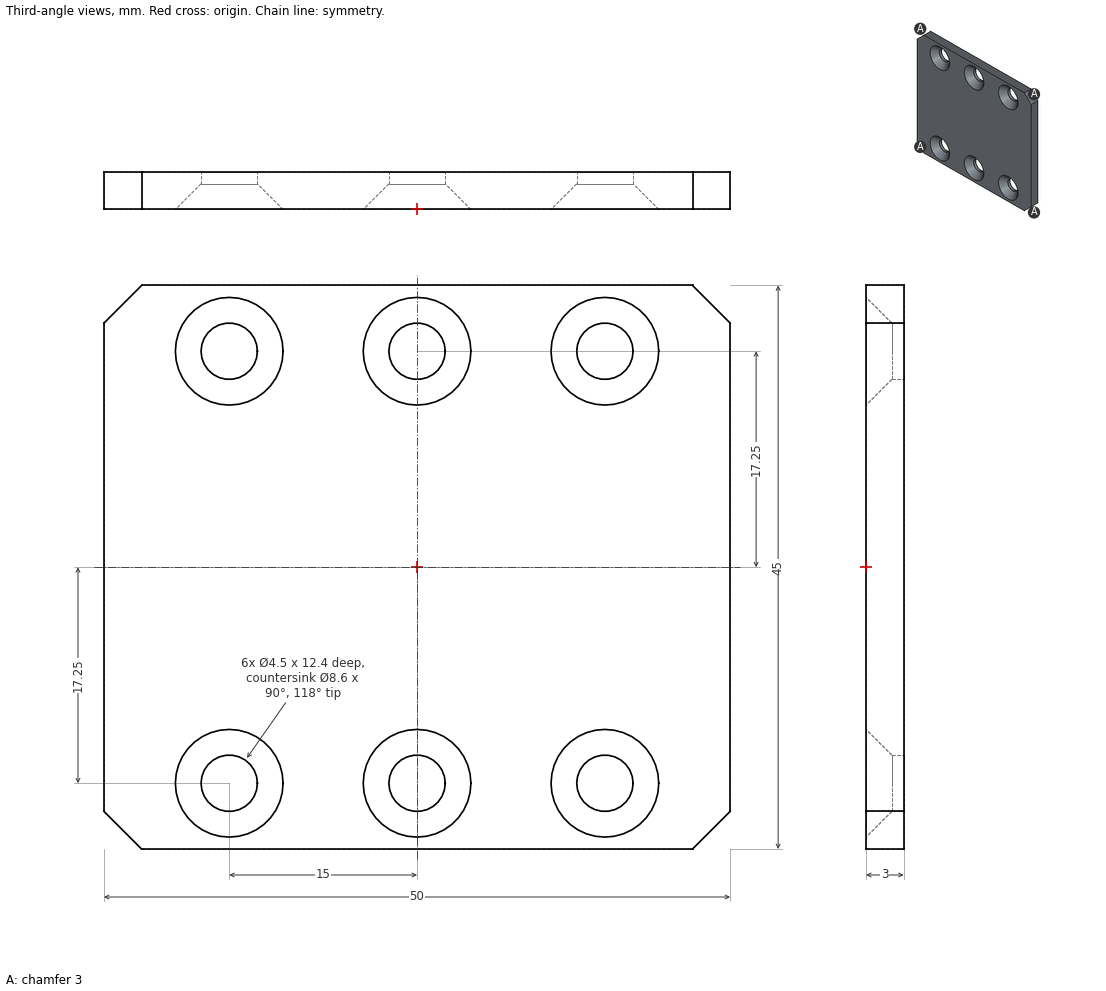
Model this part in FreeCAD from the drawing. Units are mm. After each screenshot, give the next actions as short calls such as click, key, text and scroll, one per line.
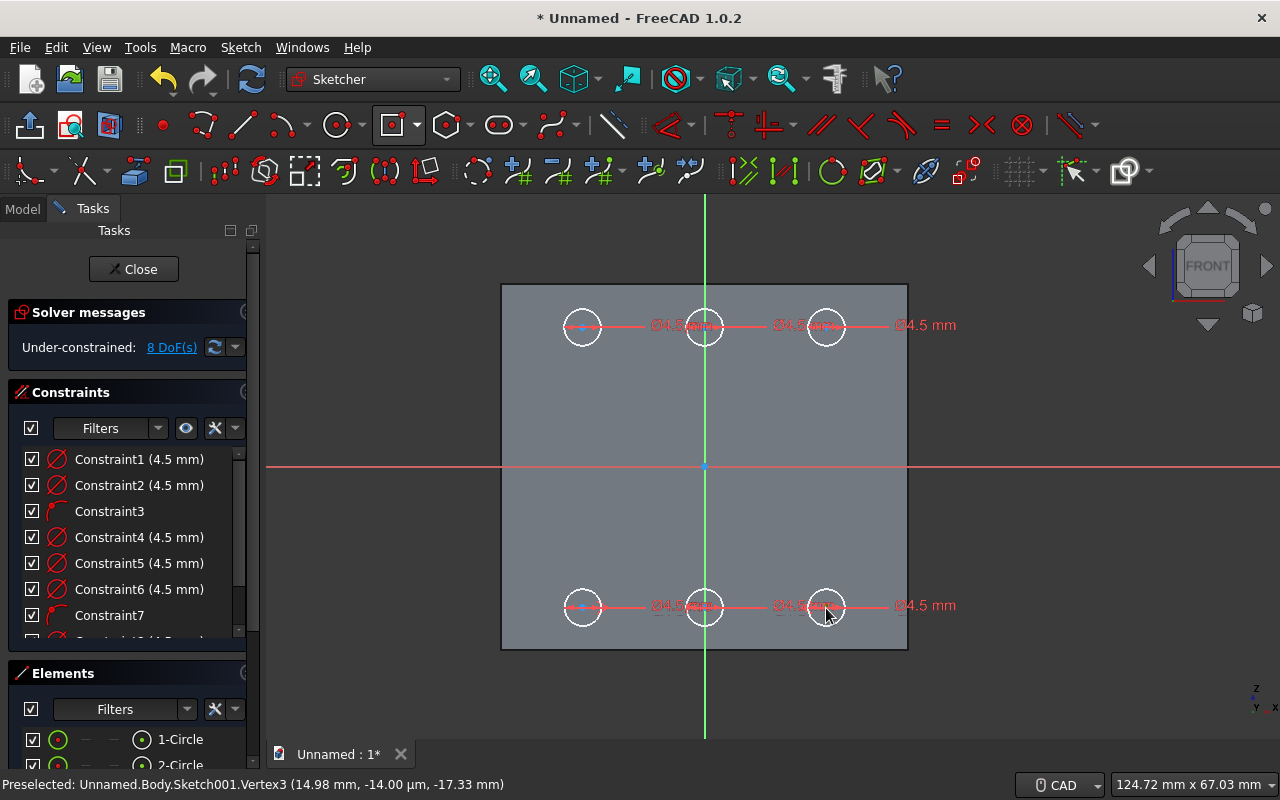
click(827, 327)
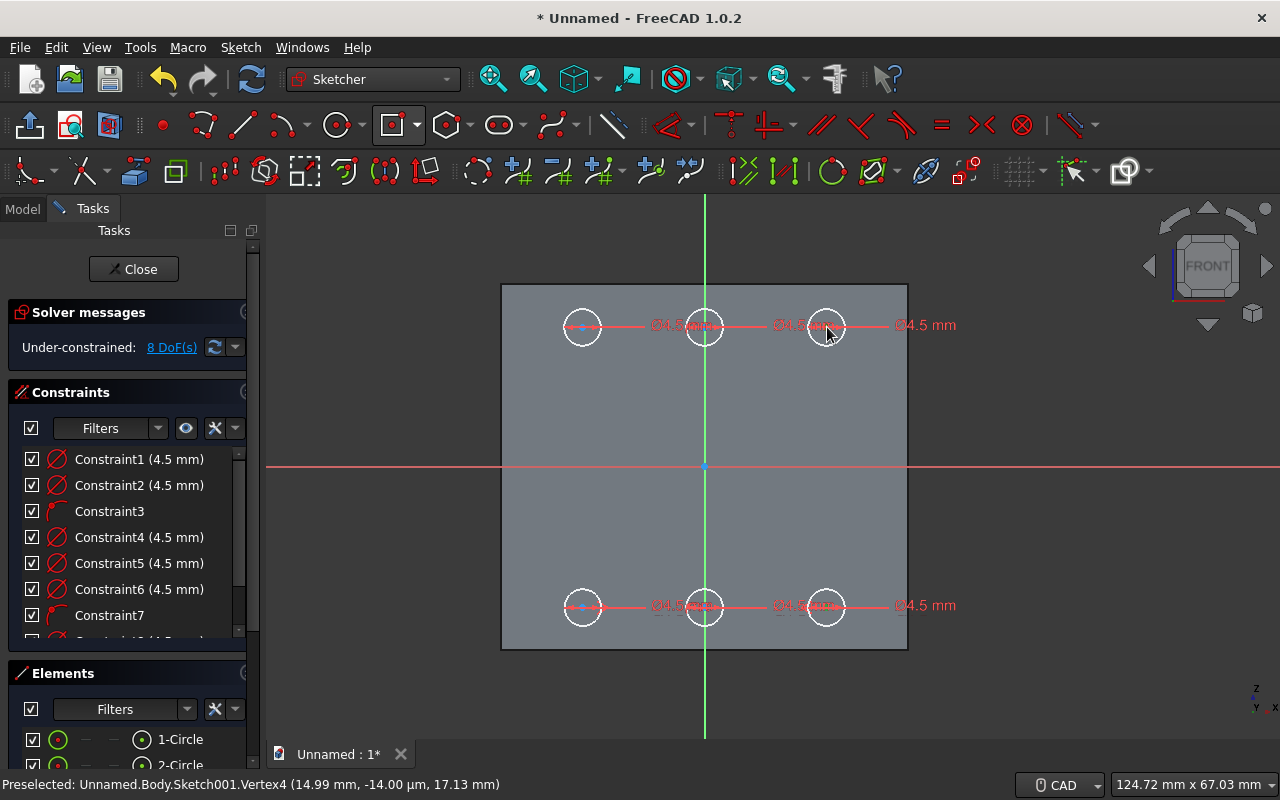
click(353, 467)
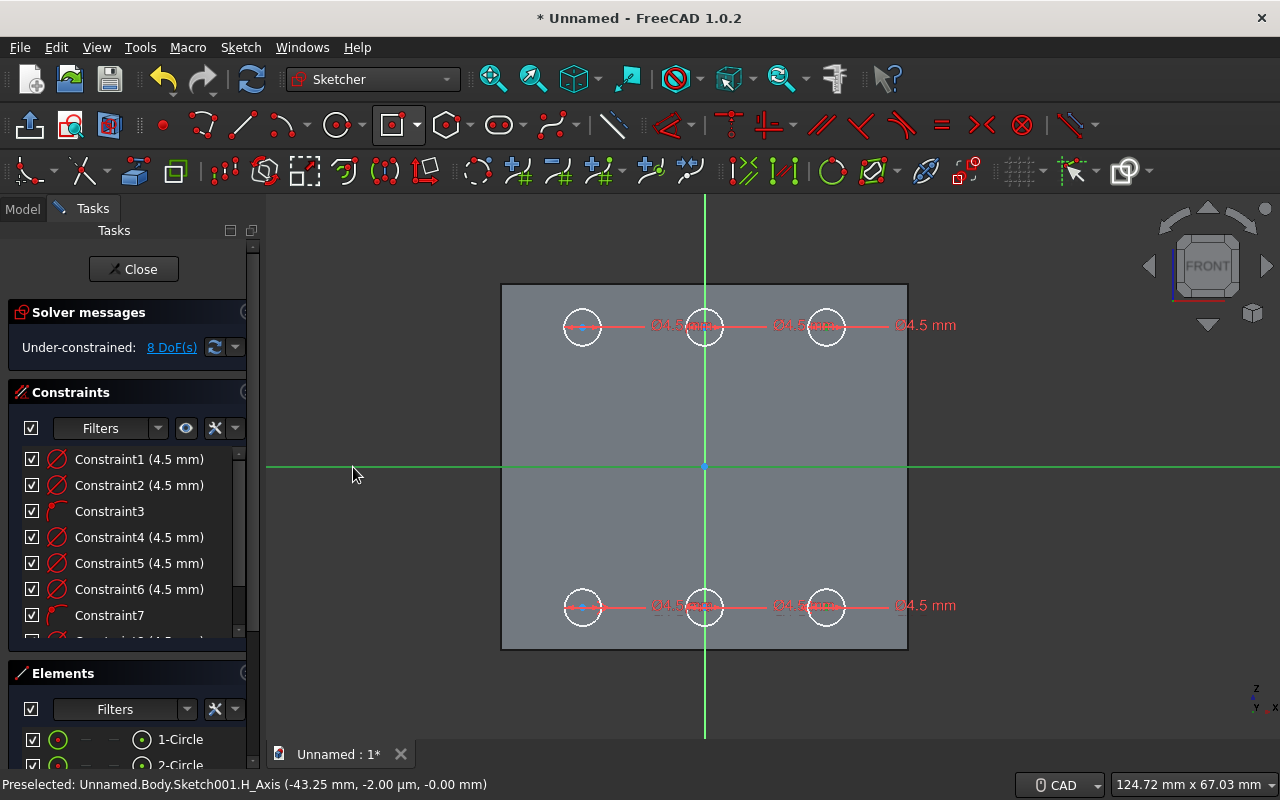
click(982, 126)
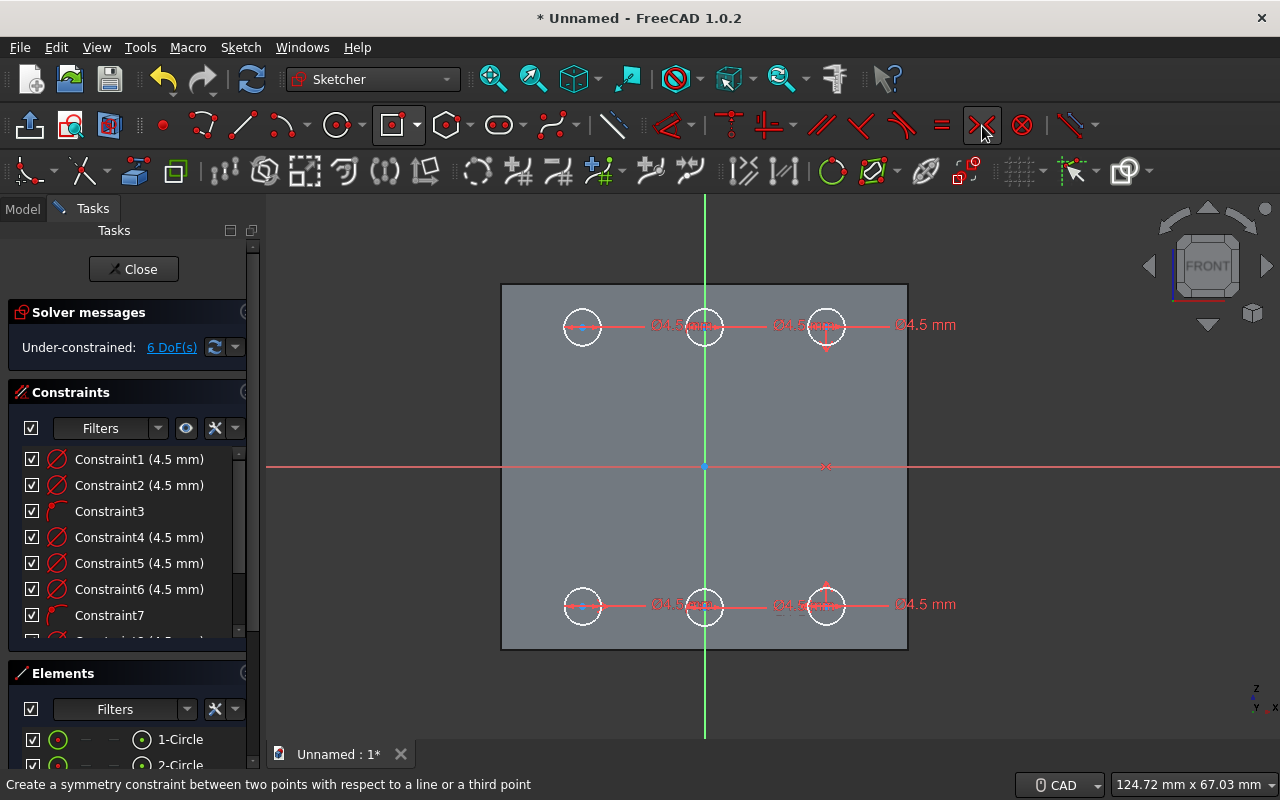
click(583, 606)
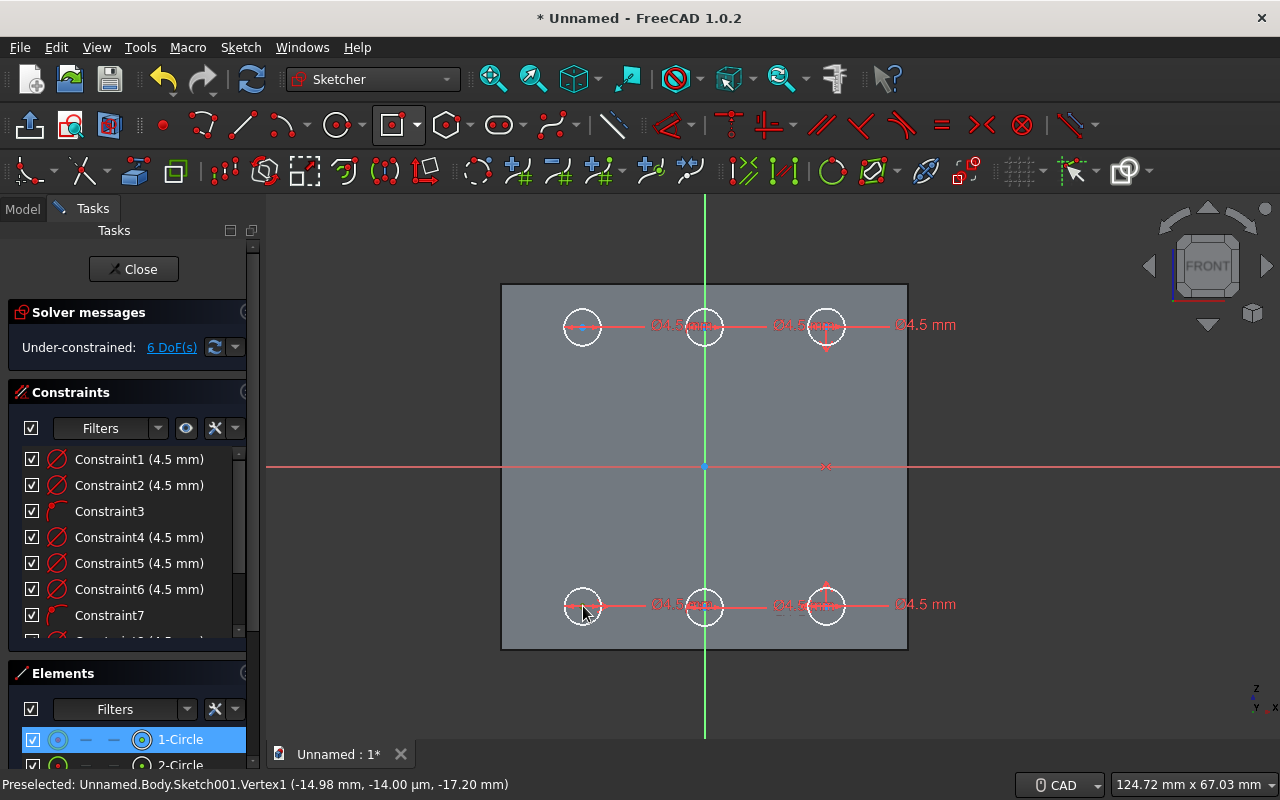
click(583, 327)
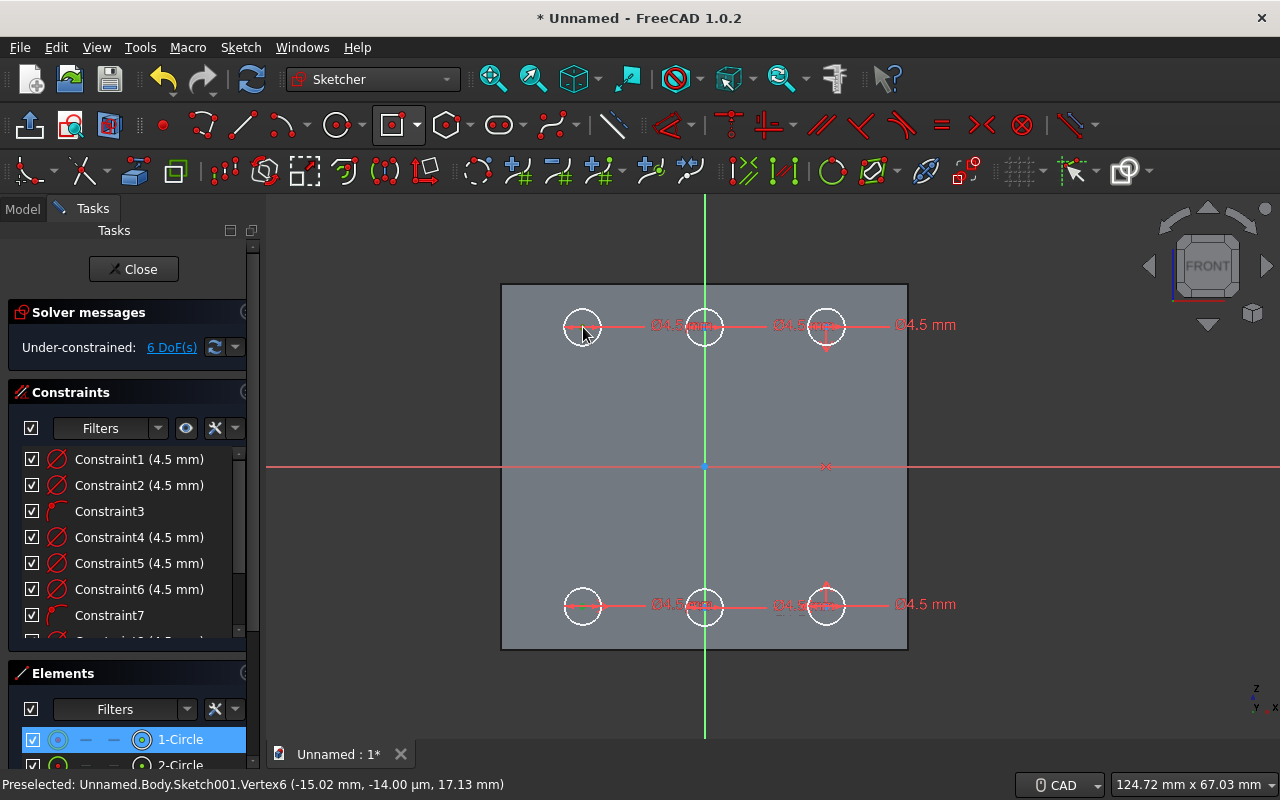
click(353, 467)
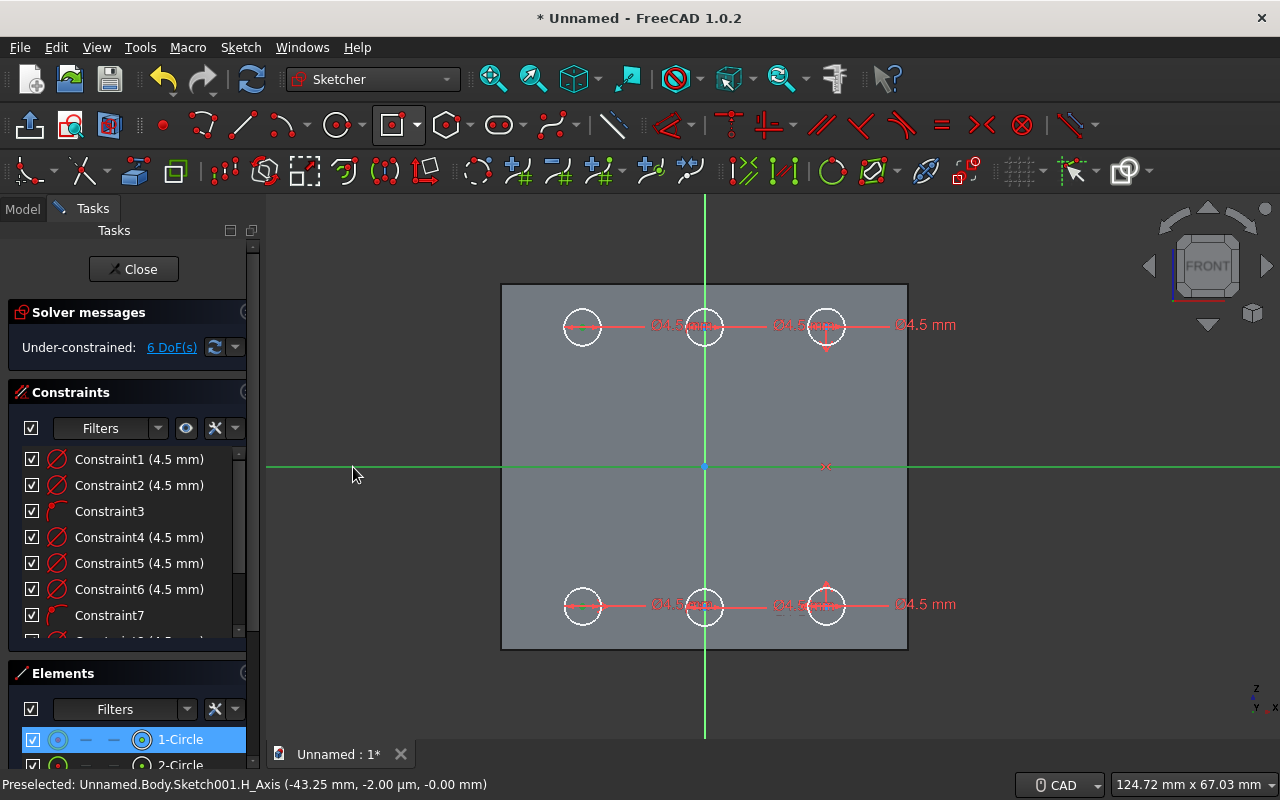
click(982, 126)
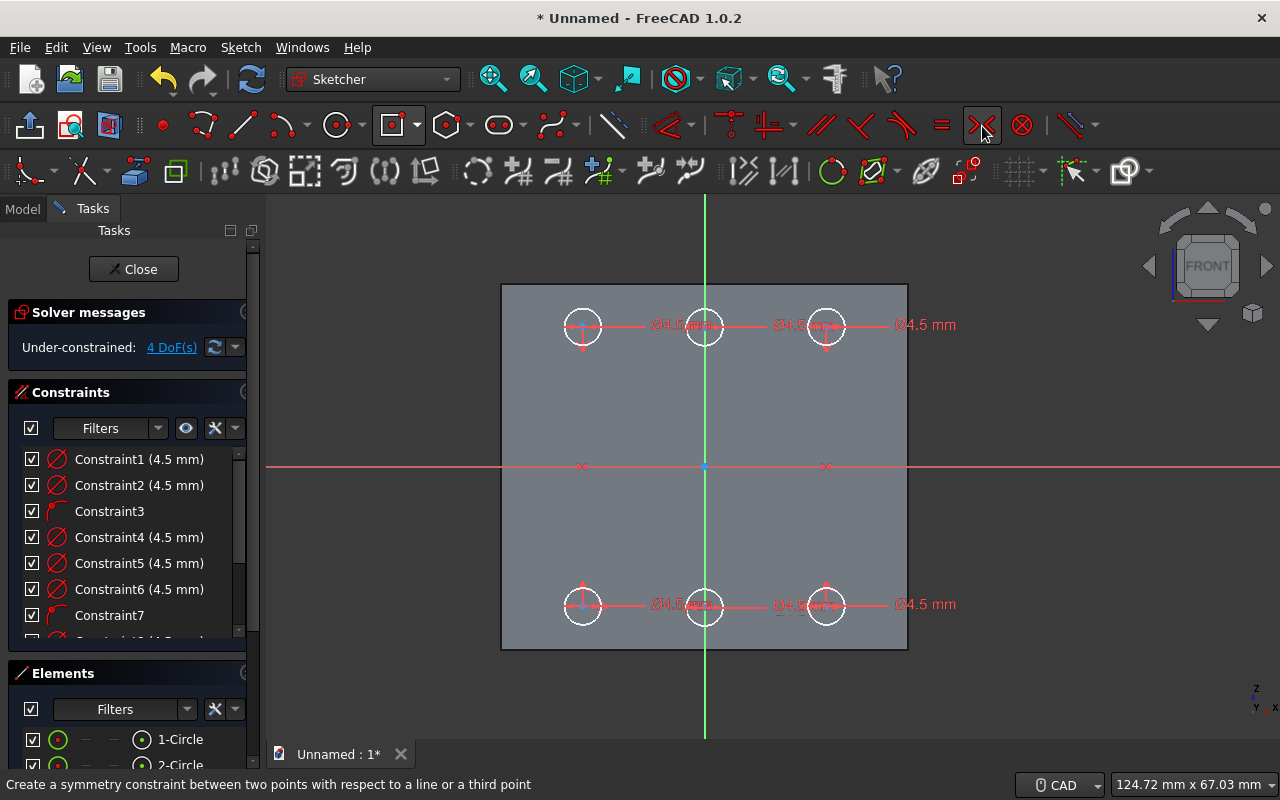
click(668, 126)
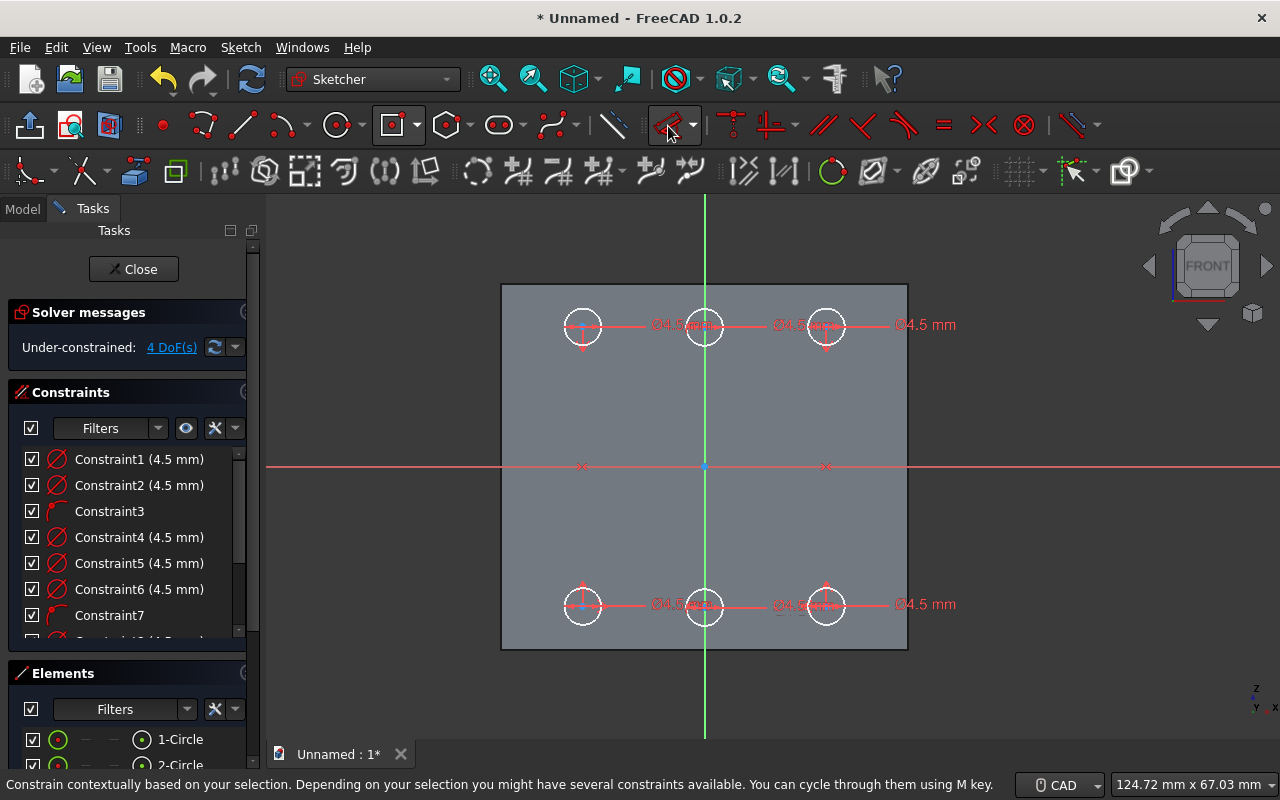
click(583, 606)
click(644, 640)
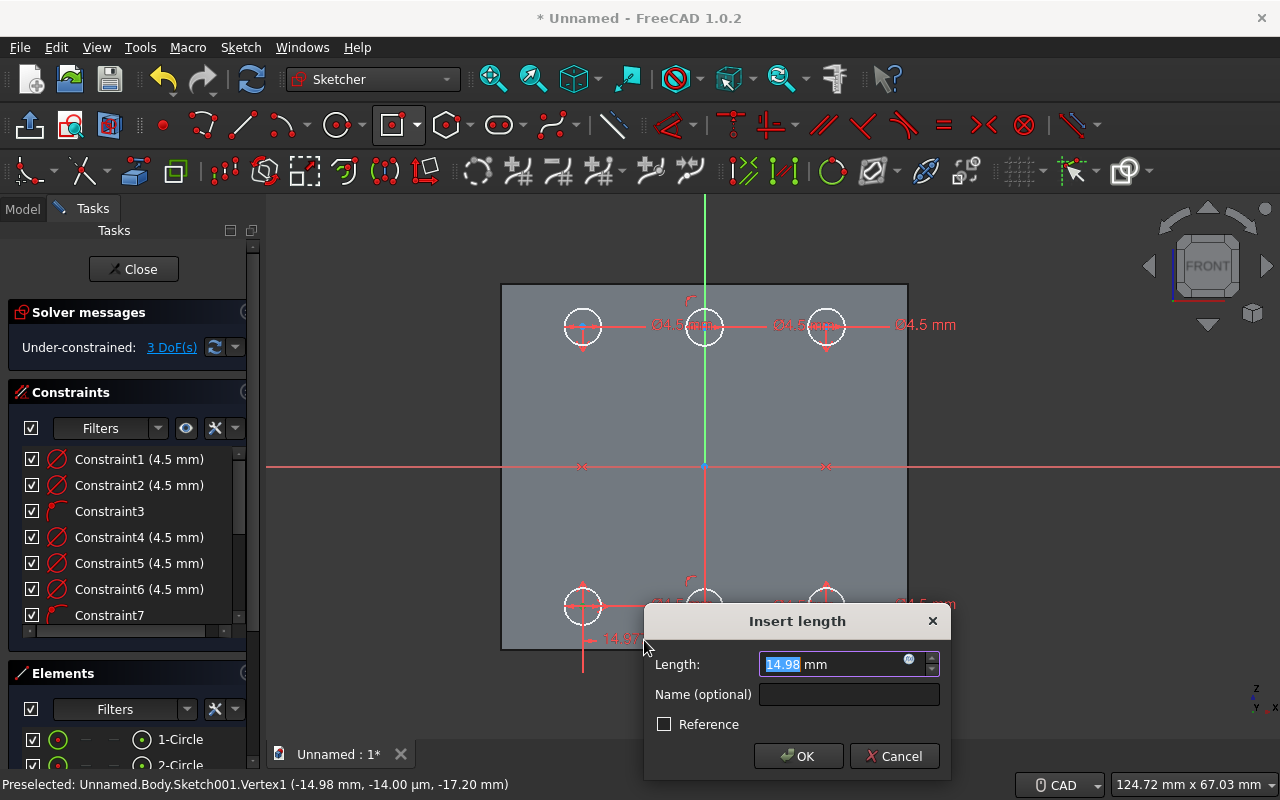
text(15)
key(Return)